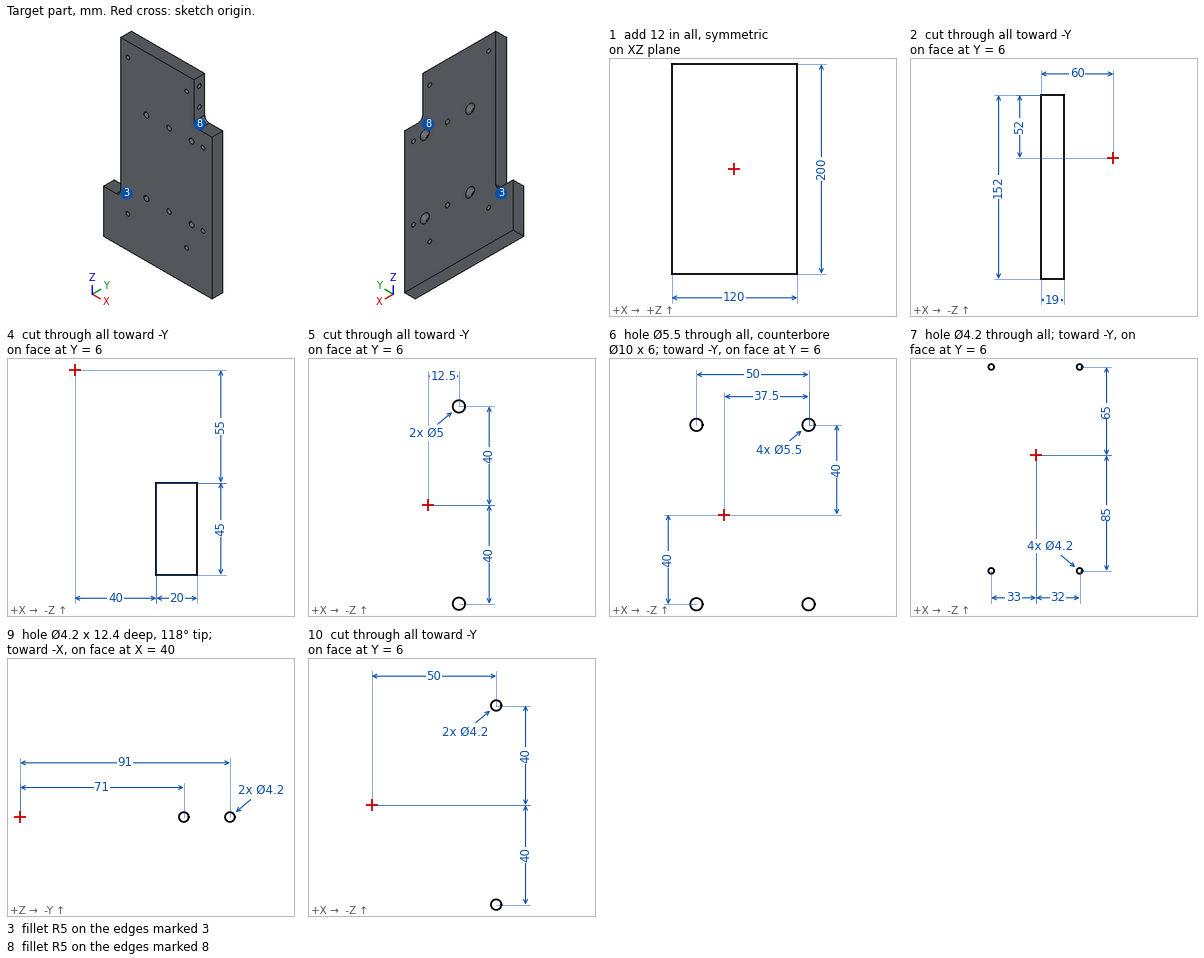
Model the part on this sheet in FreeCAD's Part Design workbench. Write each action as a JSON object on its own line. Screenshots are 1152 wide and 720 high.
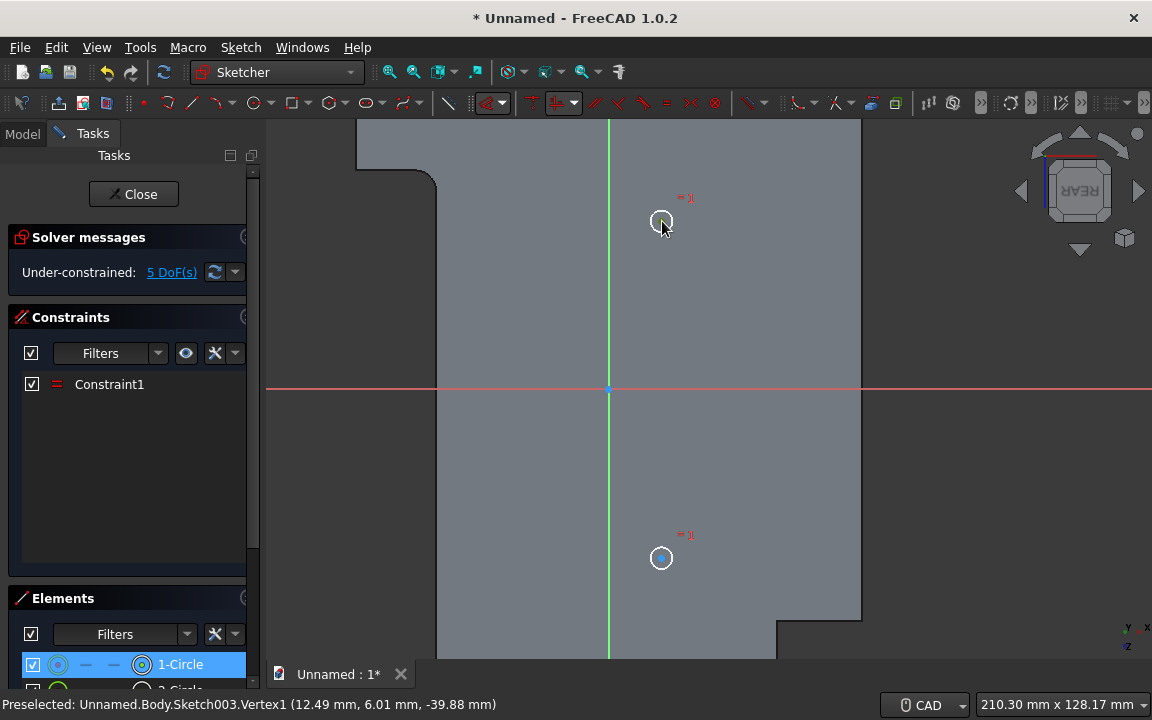
{"action": "left_click", "coordinate": [661, 558]}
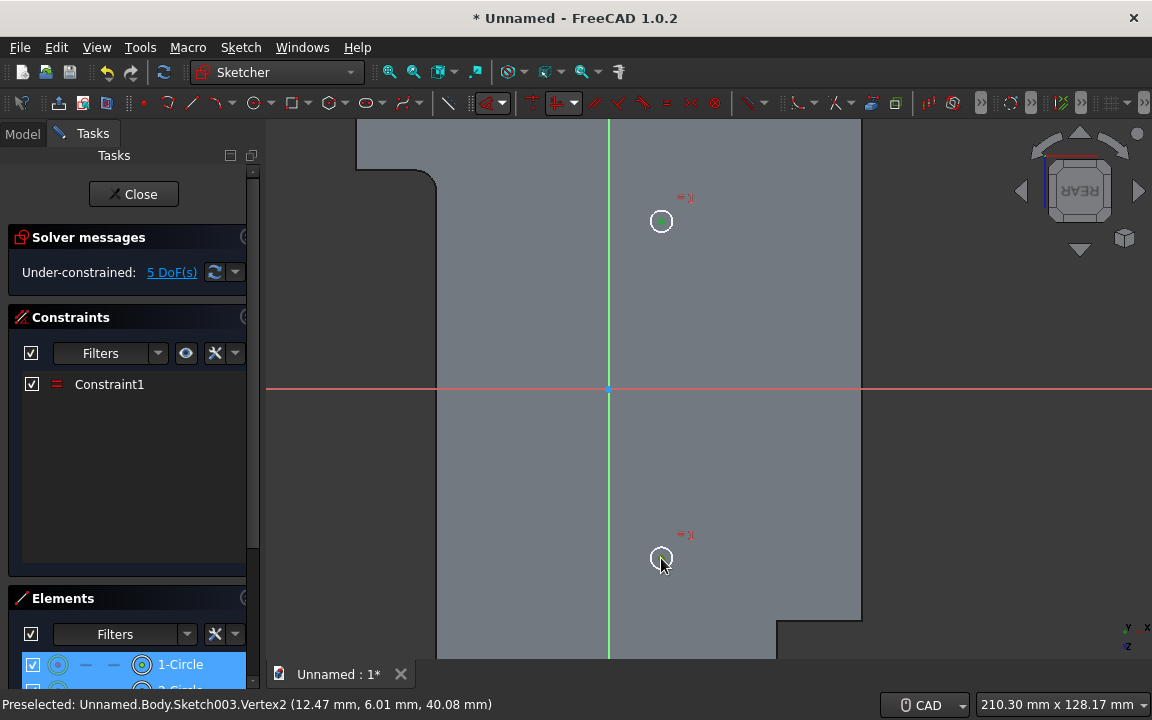
{"action": "left_click", "coordinate": [576, 104]}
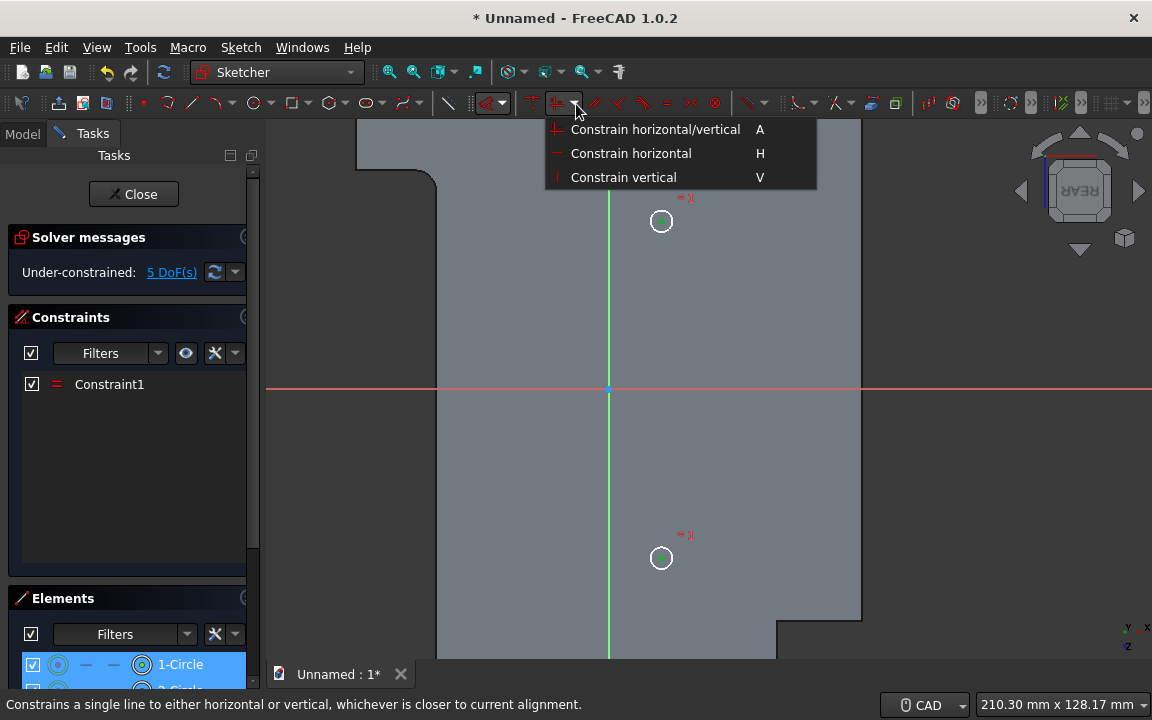
{"action": "left_click", "coordinate": [681, 177]}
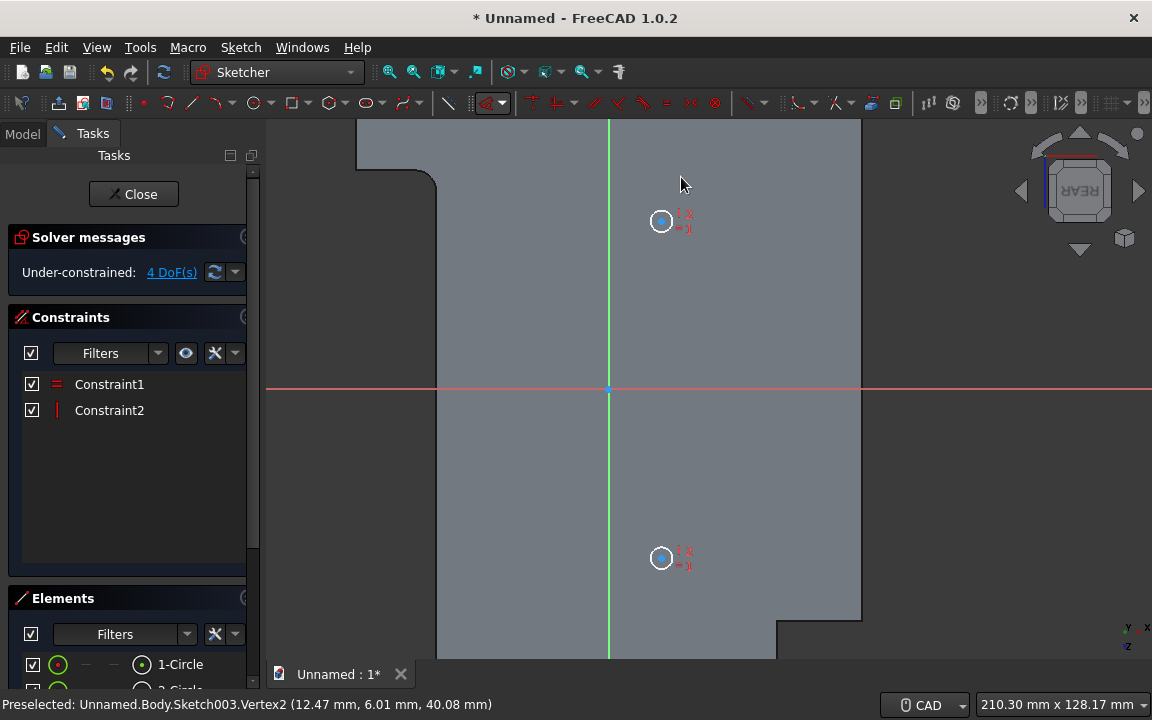
{"action": "scroll", "coordinate": [669, 214], "scroll_direction": "up", "scroll_amount": 4}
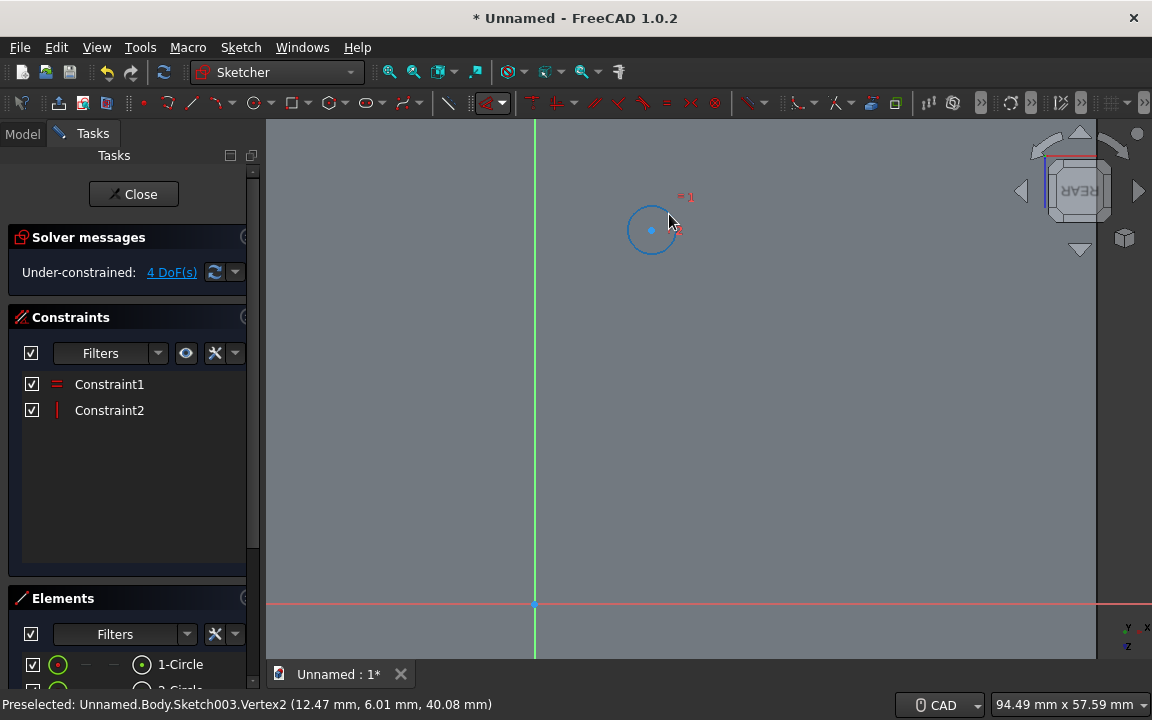
{"action": "left_click", "coordinate": [669, 213]}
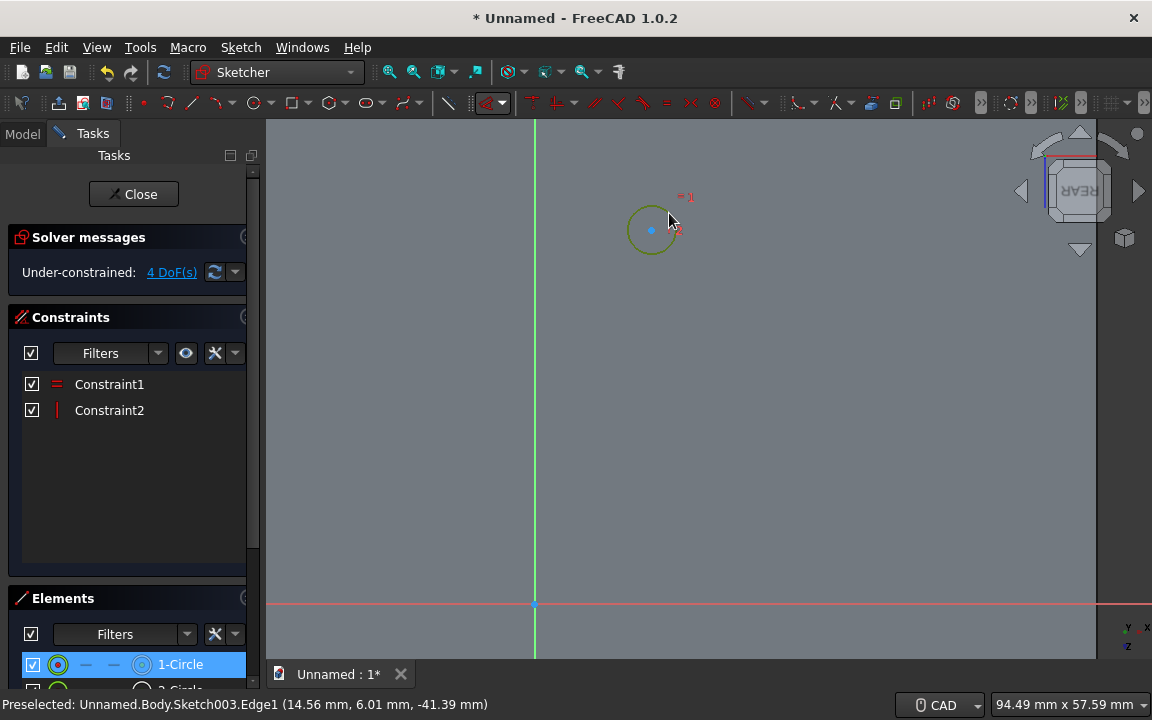
{"action": "left_click", "coordinate": [504, 104]}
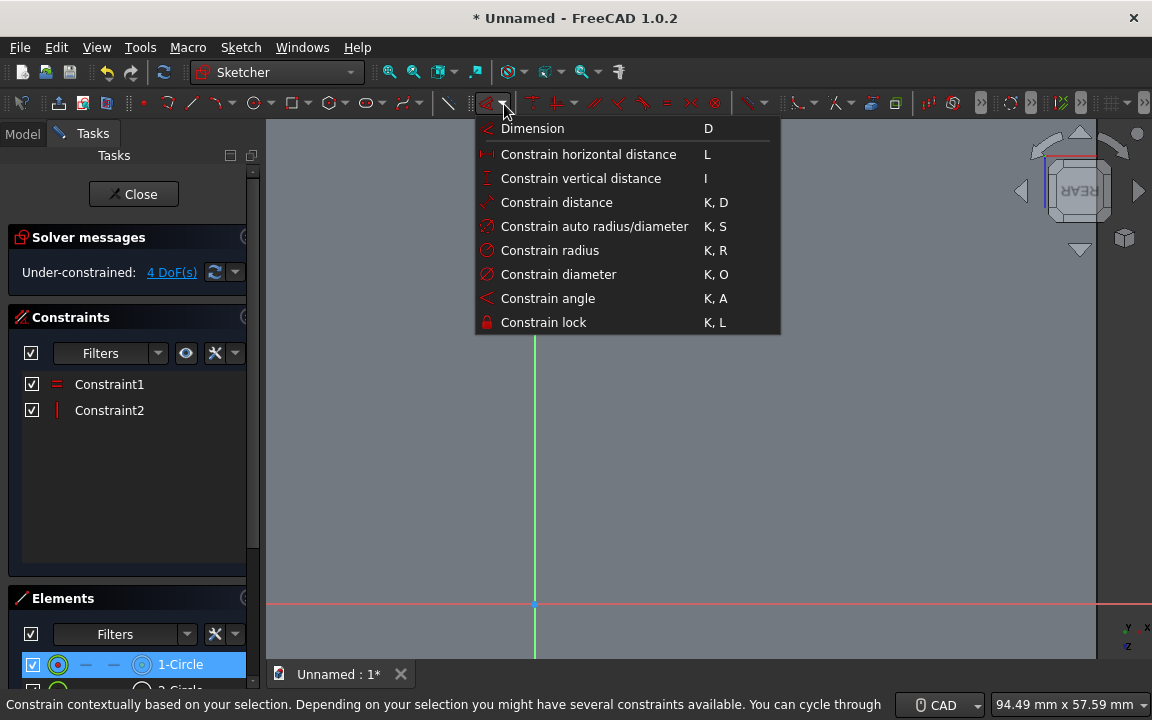
{"action": "left_click", "coordinate": [628, 274]}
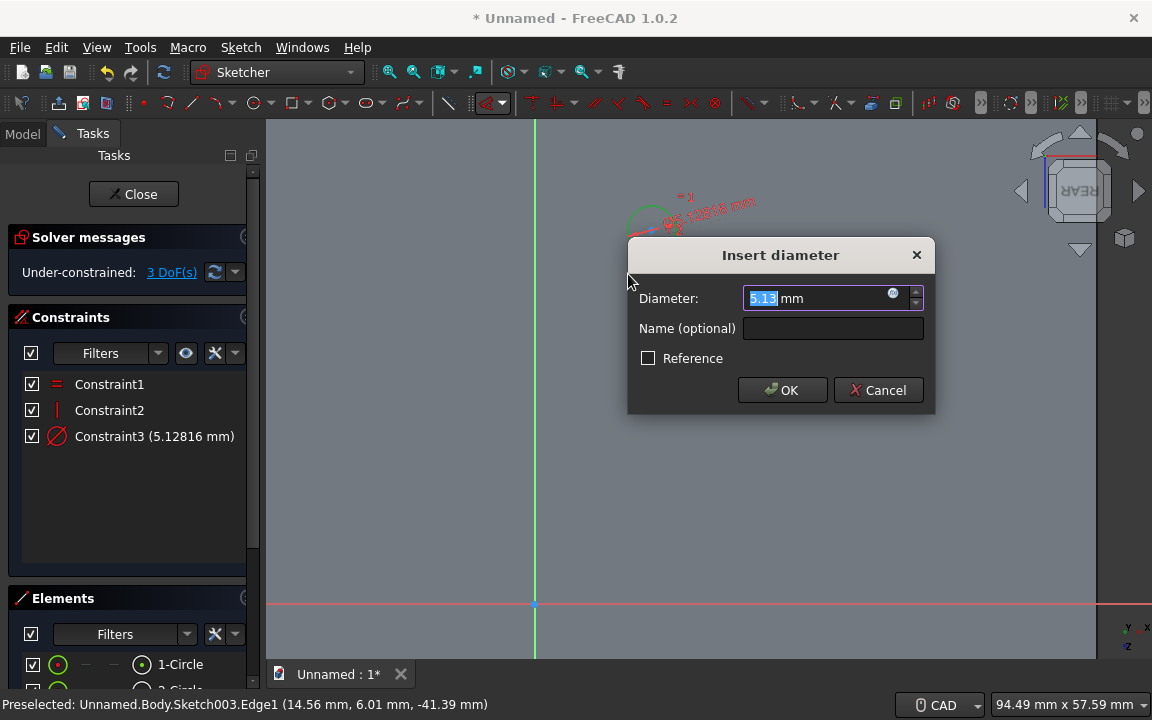
{"action": "type", "text": "5"}
{"action": "key", "text": "Return"}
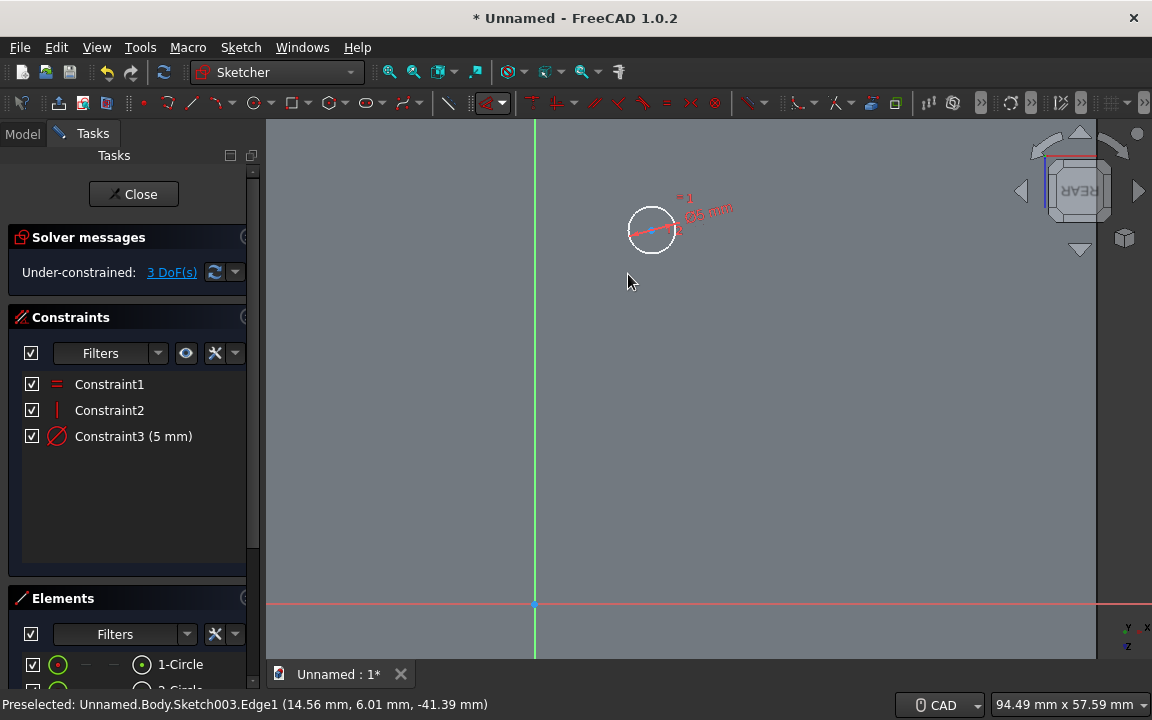
{"action": "left_click", "coordinate": [652, 230]}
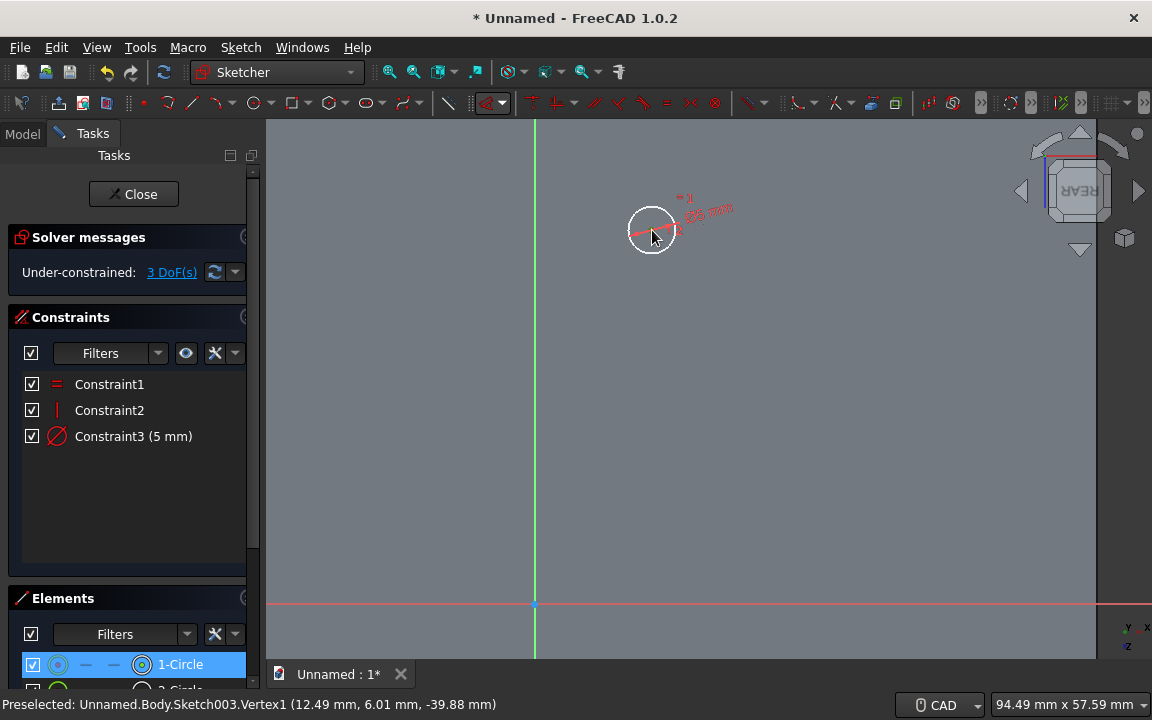
{"action": "key", "text": "i"}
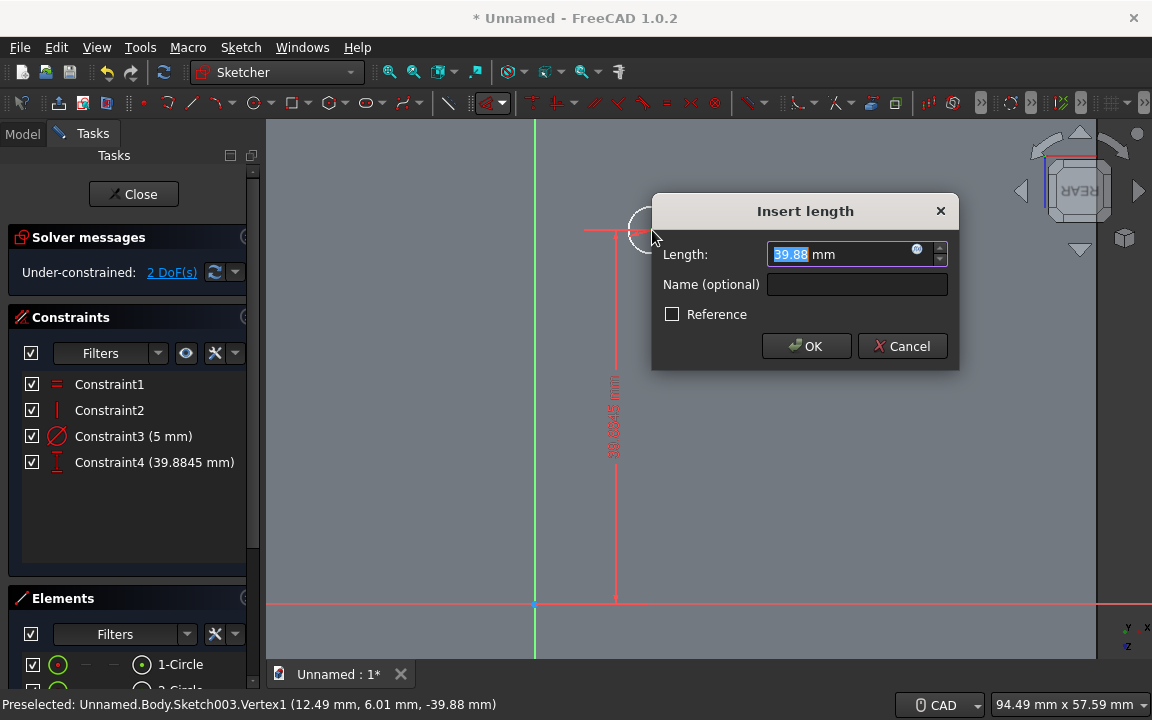
{"action": "type", "text": "40"}
{"action": "key", "text": "Return"}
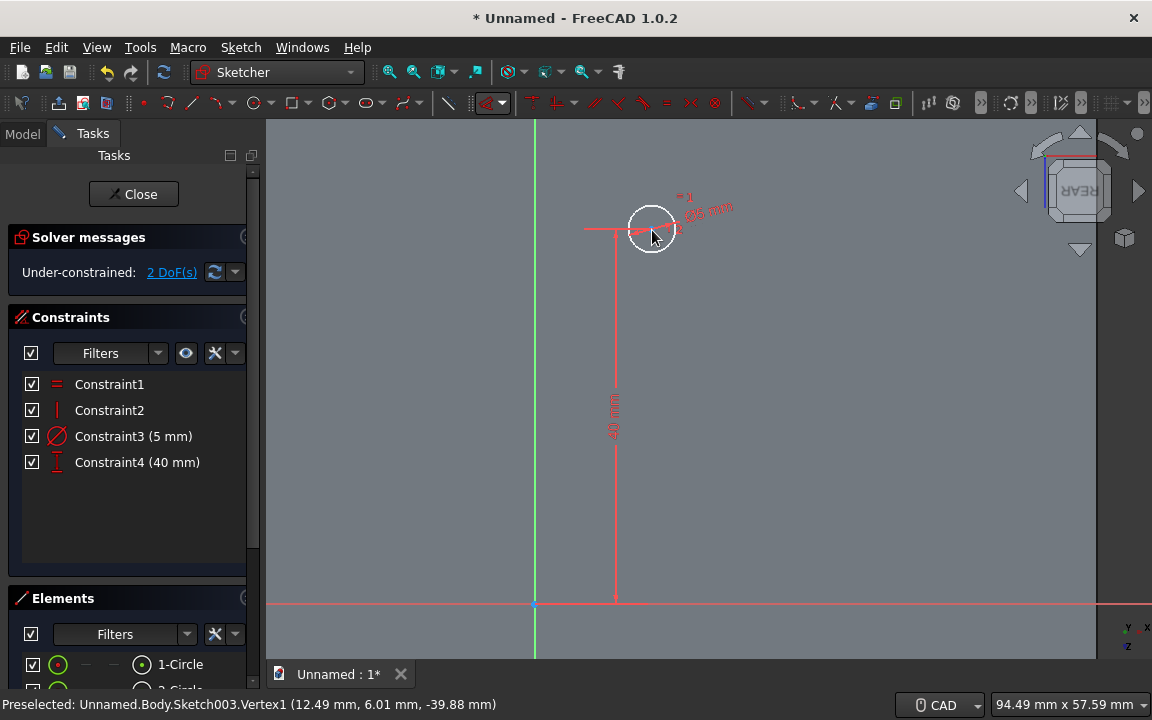
{"action": "scroll", "coordinate": [669, 214], "scroll_direction": "down", "scroll_amount": 4}